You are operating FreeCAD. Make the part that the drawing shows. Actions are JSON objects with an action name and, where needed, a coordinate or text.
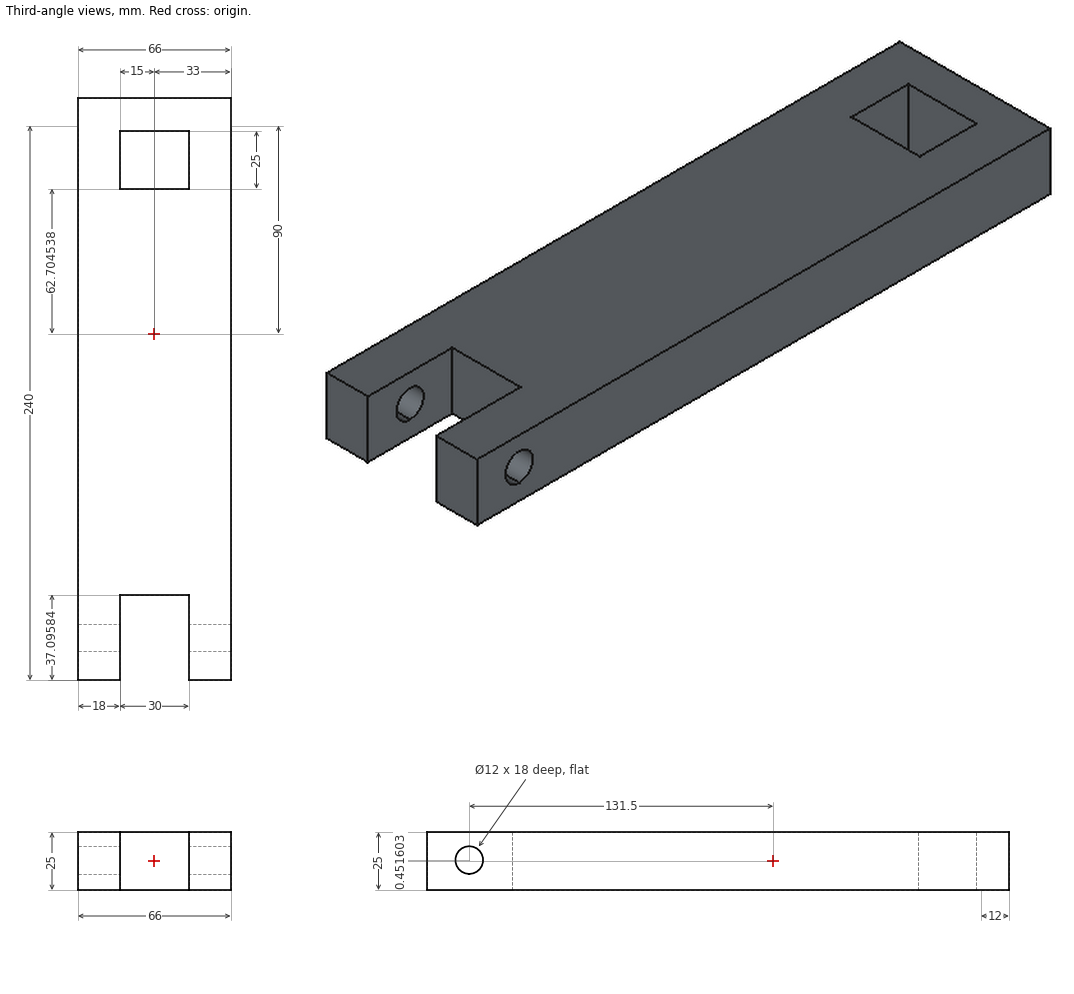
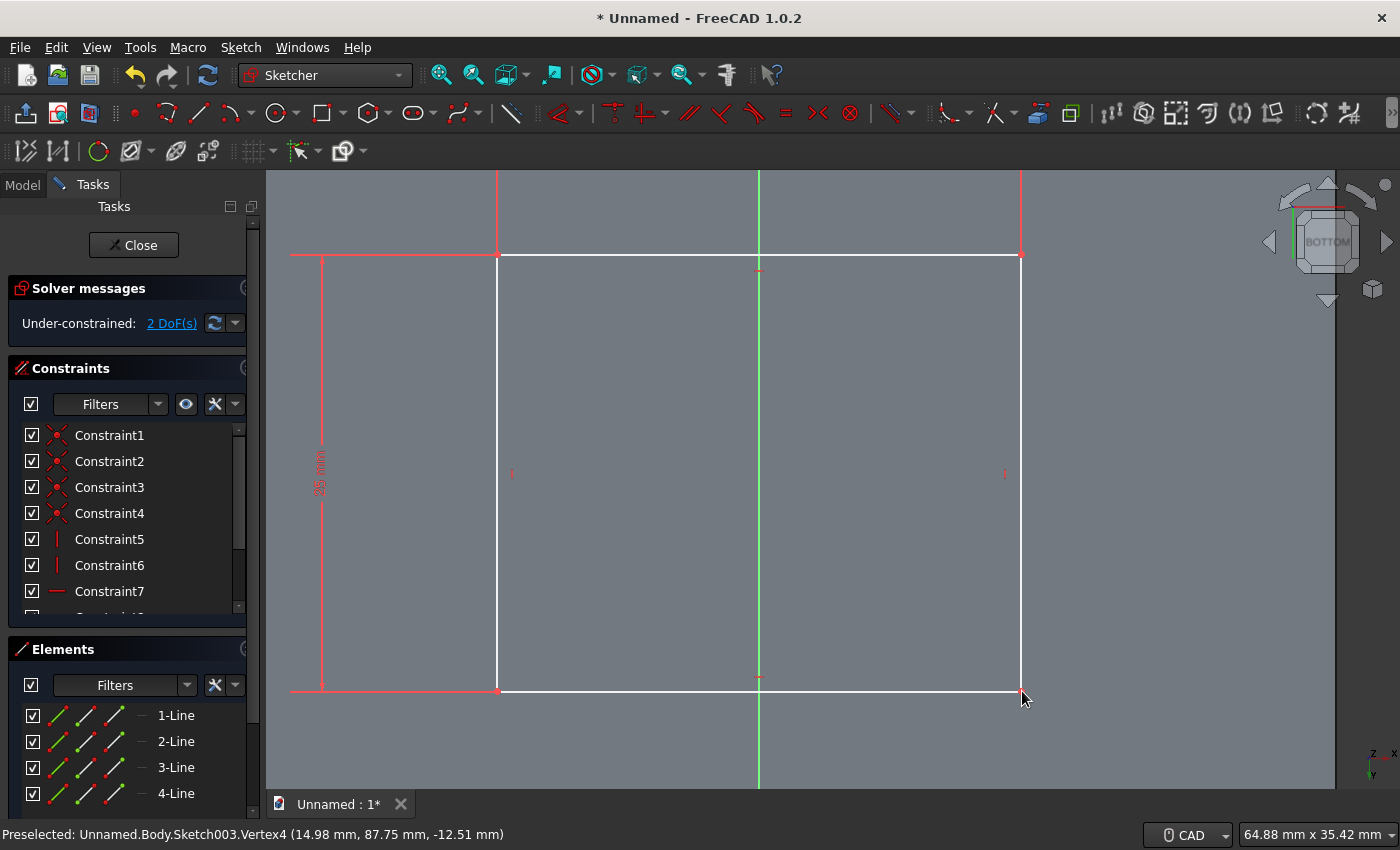
{"action": "left_click", "coordinate": [558, 114]}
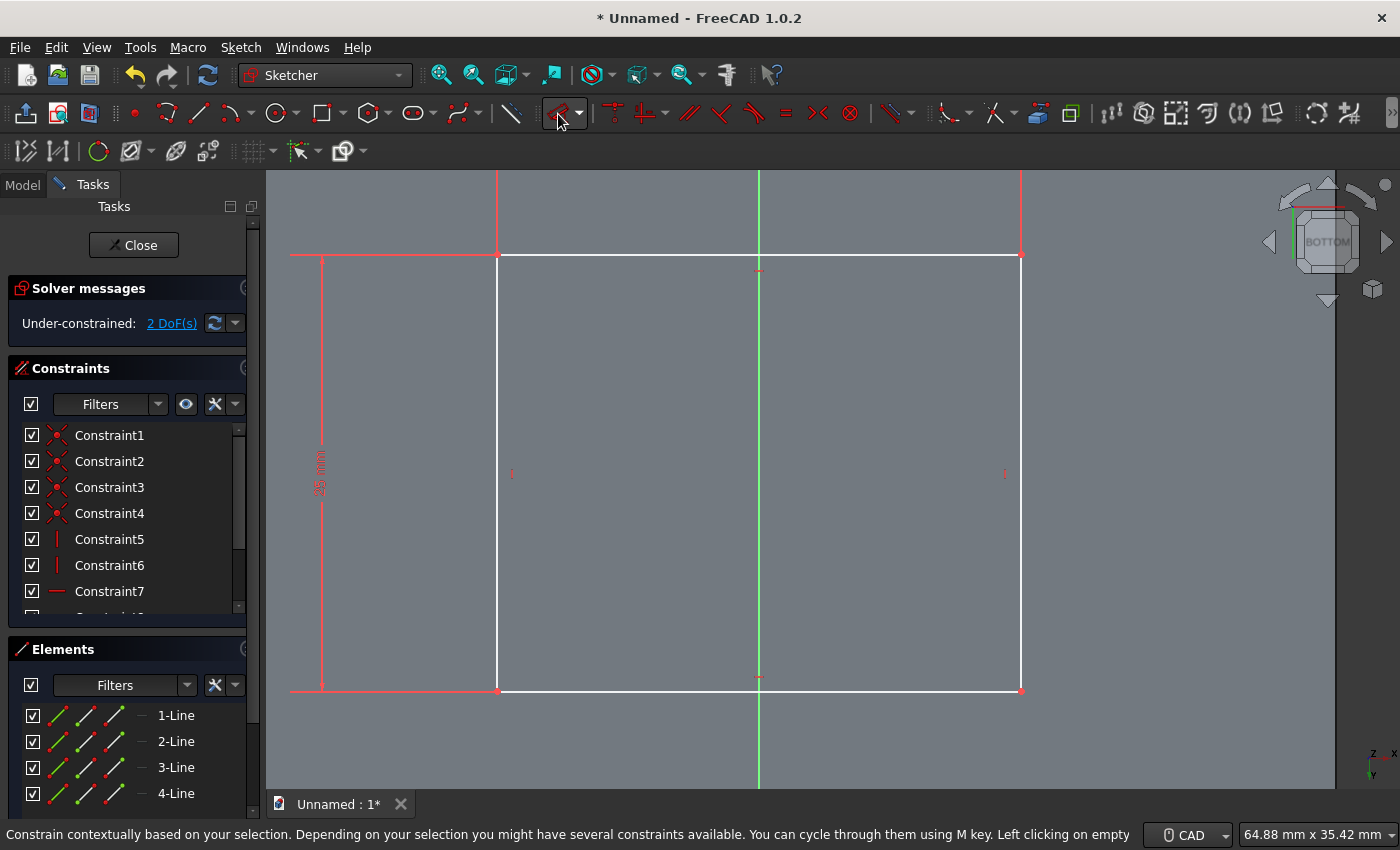
{"action": "left_click", "coordinate": [497, 255]}
{"action": "left_click", "coordinate": [628, 289]}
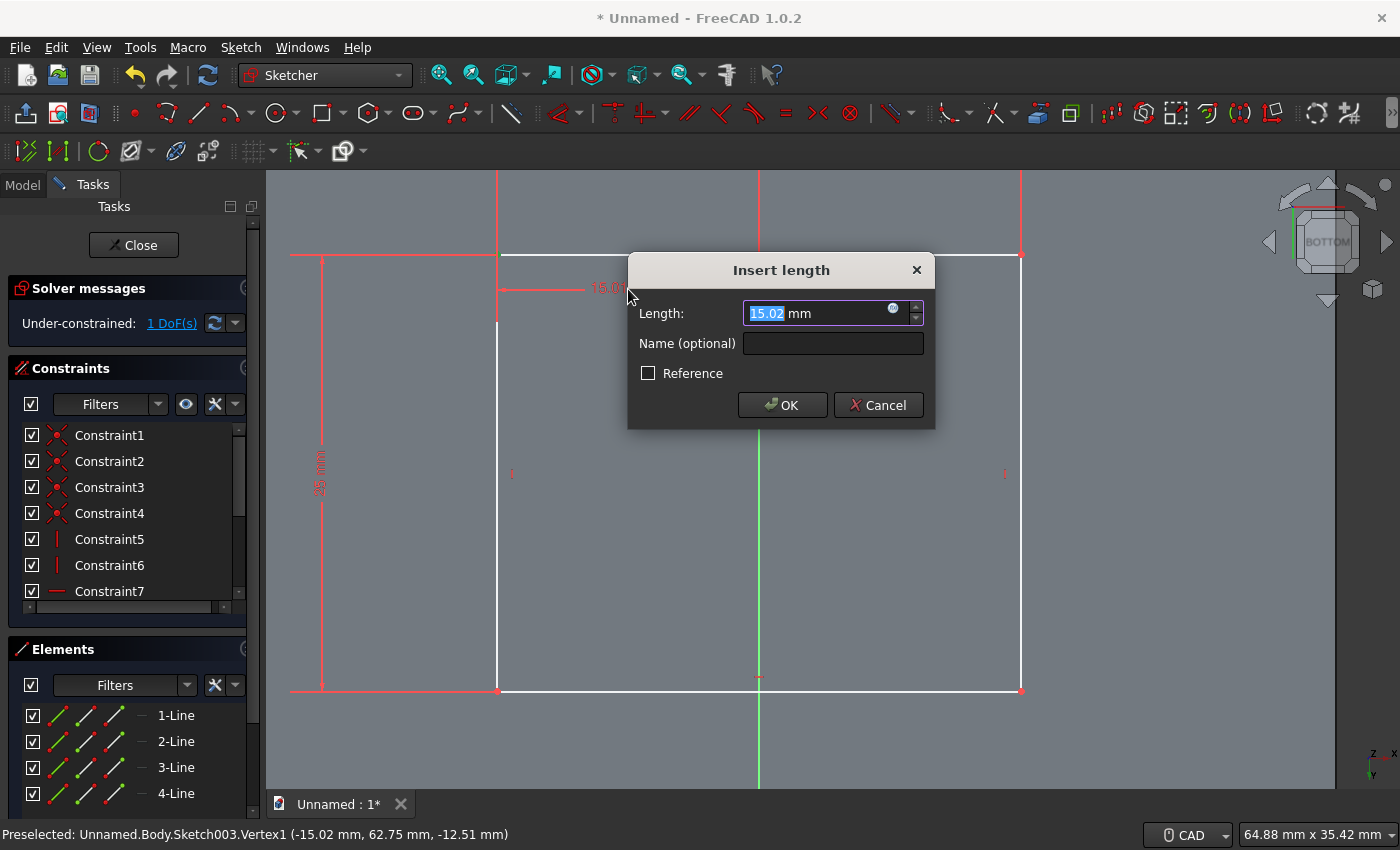
{"action": "type", "text": "15"}
{"action": "key", "text": "Return"}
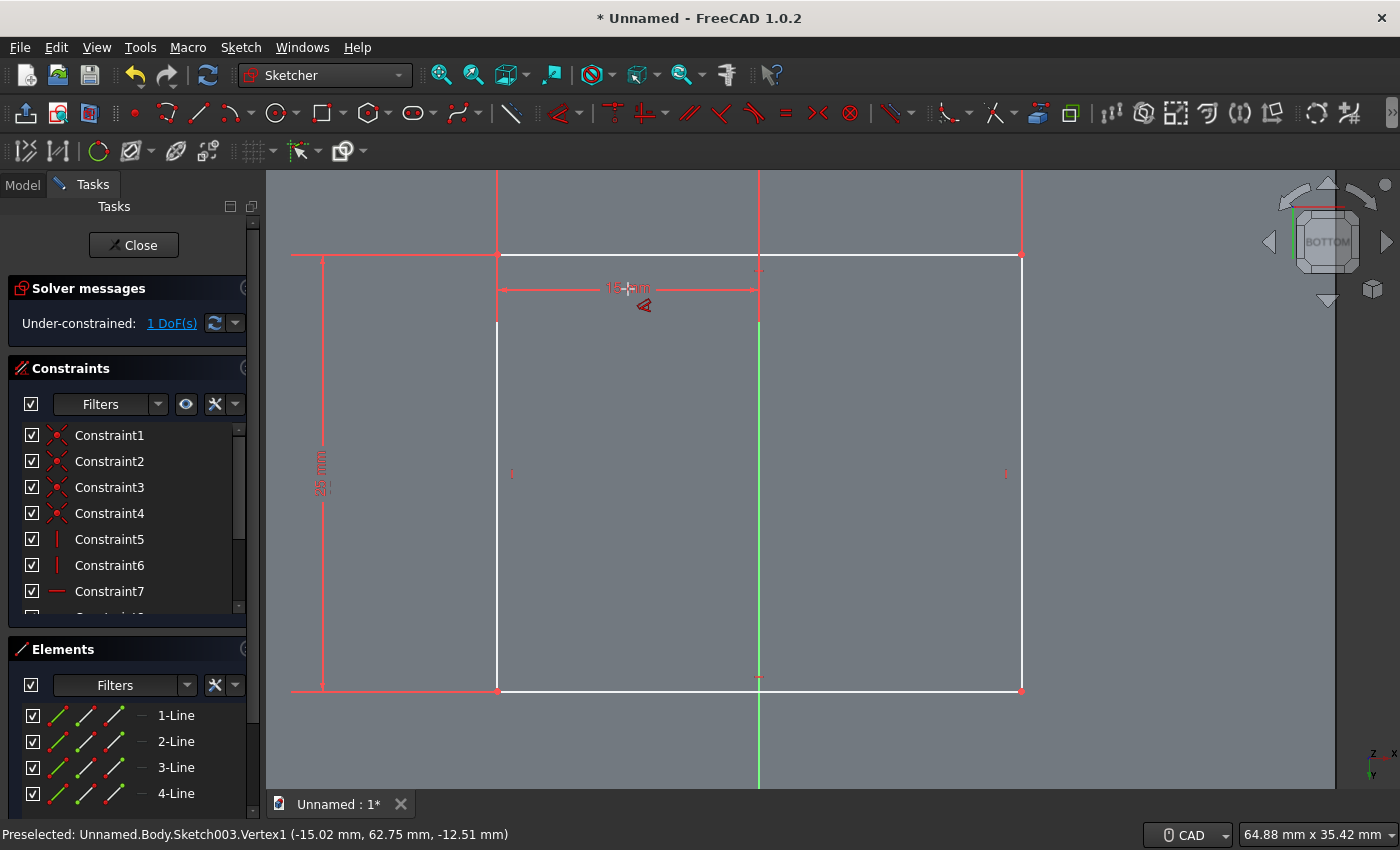
{"action": "left_click", "coordinate": [497, 255]}
{"action": "left_click", "coordinate": [463, 226]}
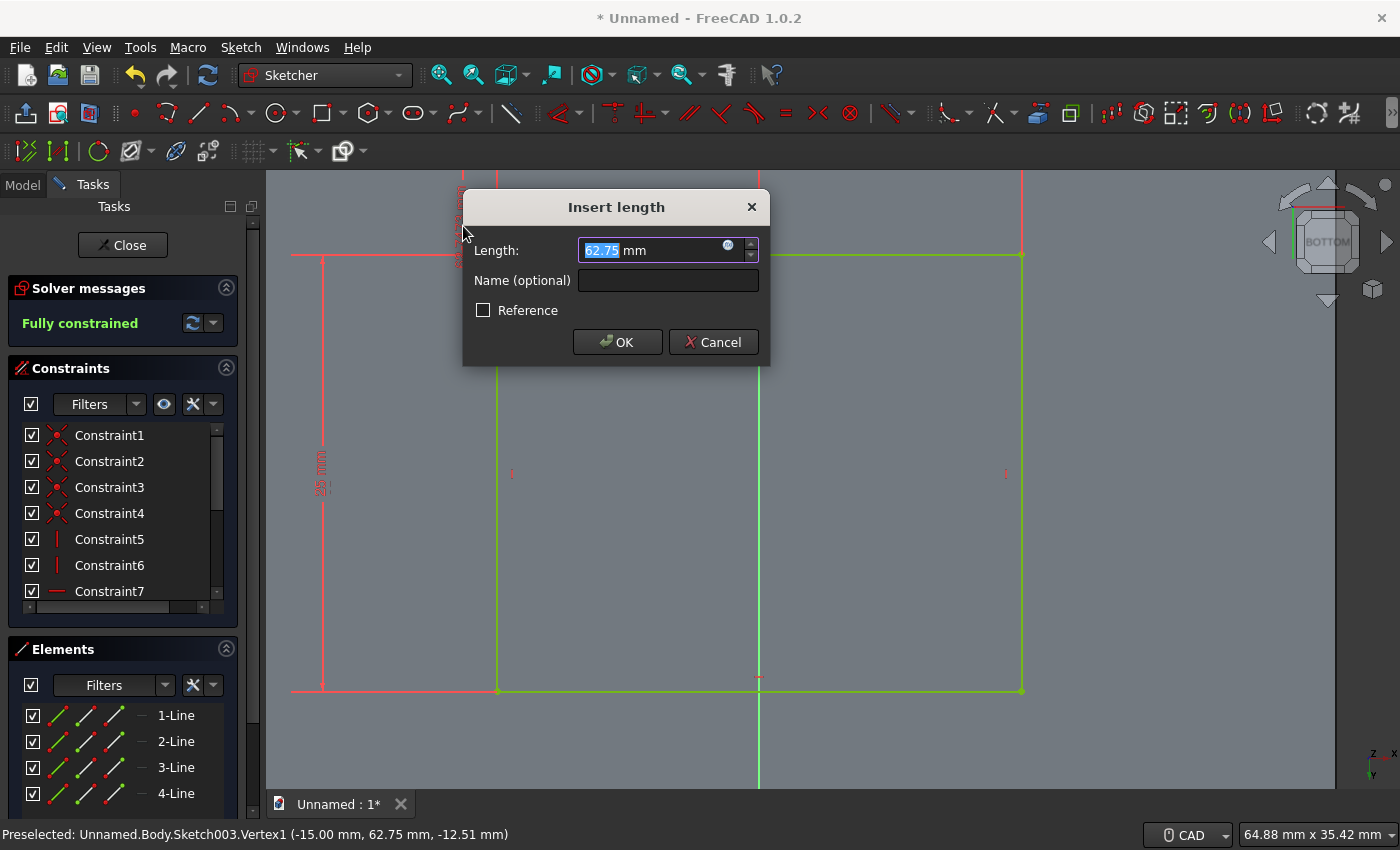
{"action": "type", "text": "62.704538"}
{"action": "key", "text": "Return"}
{"action": "key", "text": "Escape"}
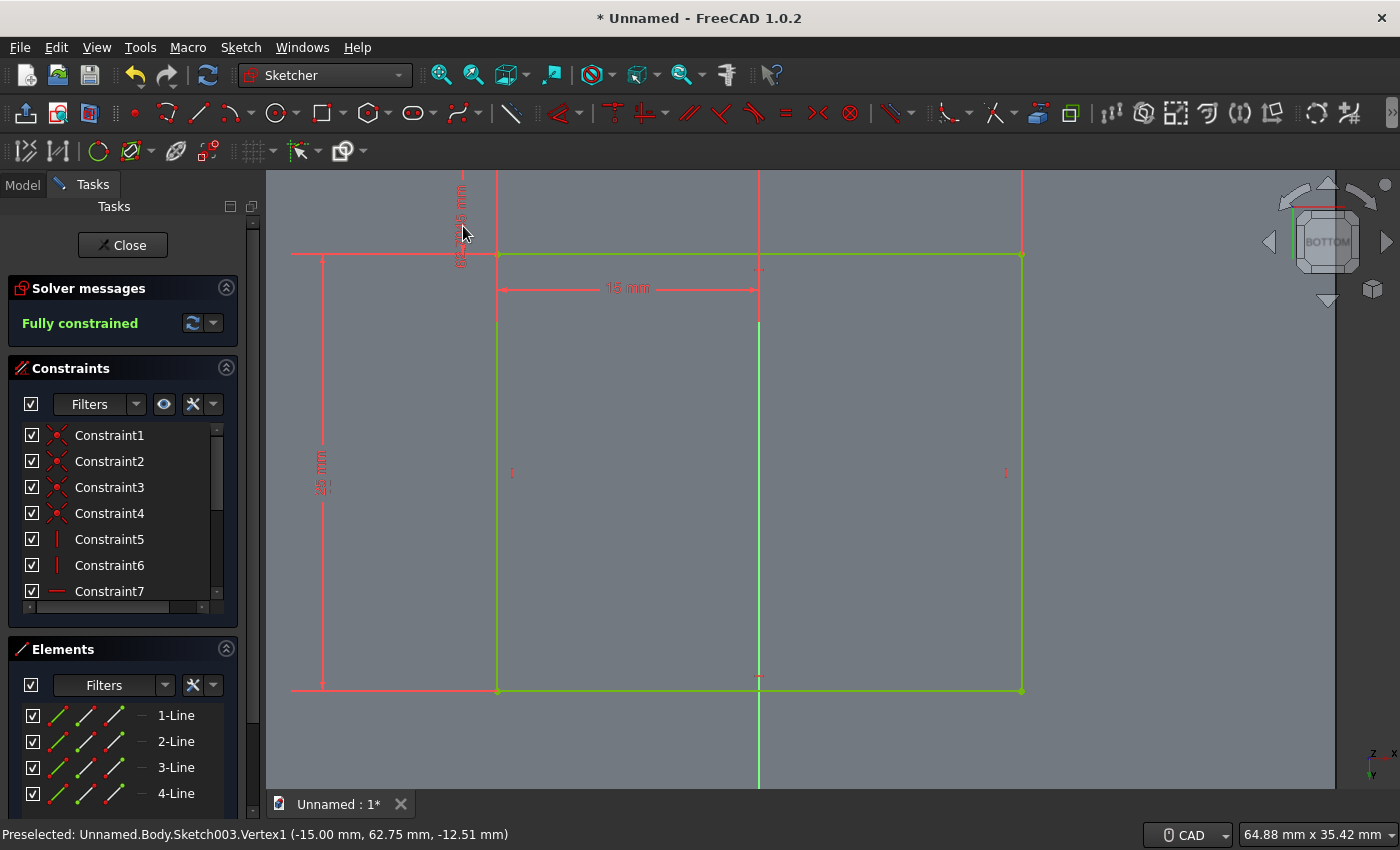
{"action": "left_click", "coordinate": [123, 245]}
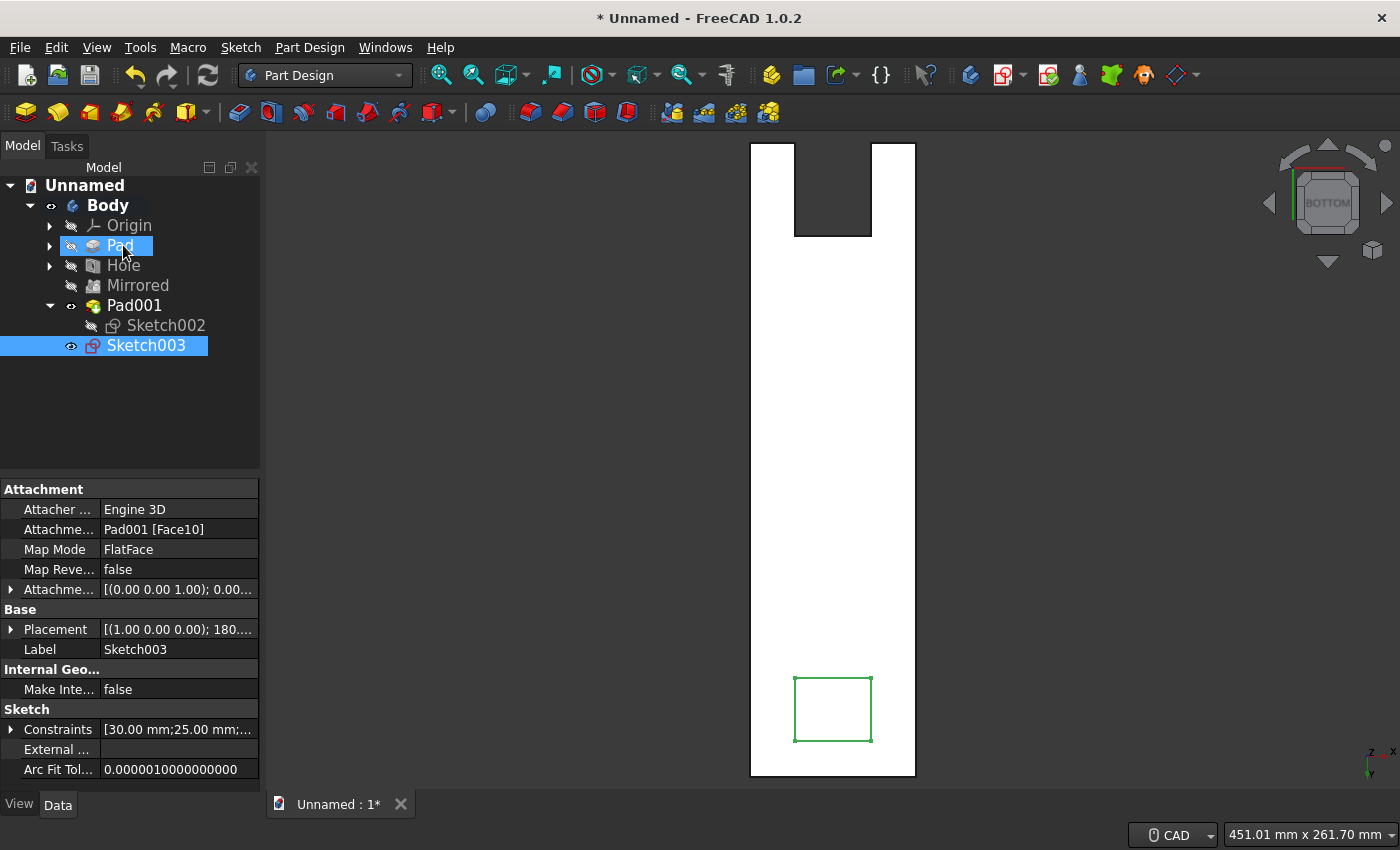
{"action": "left_click", "coordinate": [240, 112]}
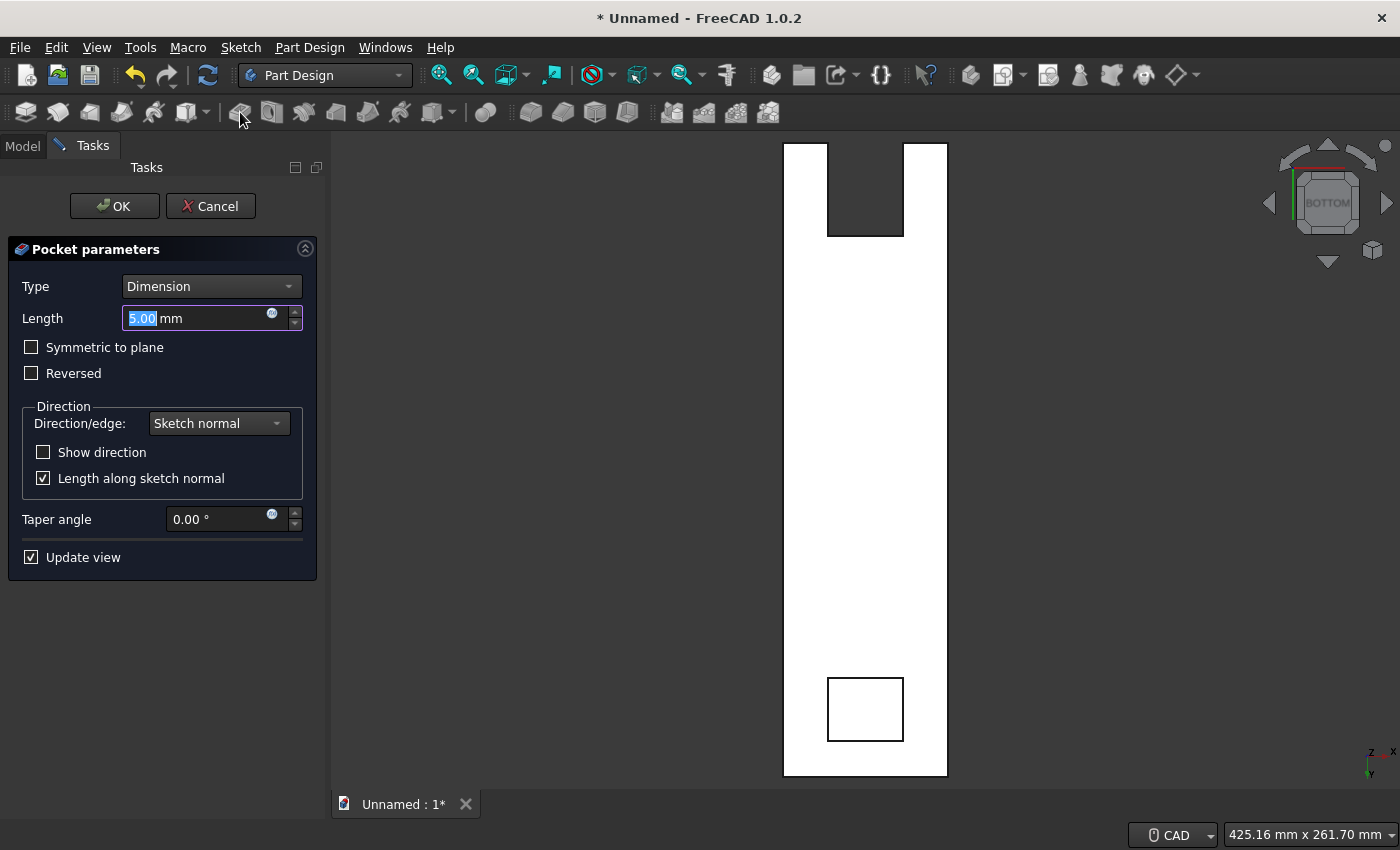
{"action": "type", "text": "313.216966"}
{"action": "key", "text": "Tab"}